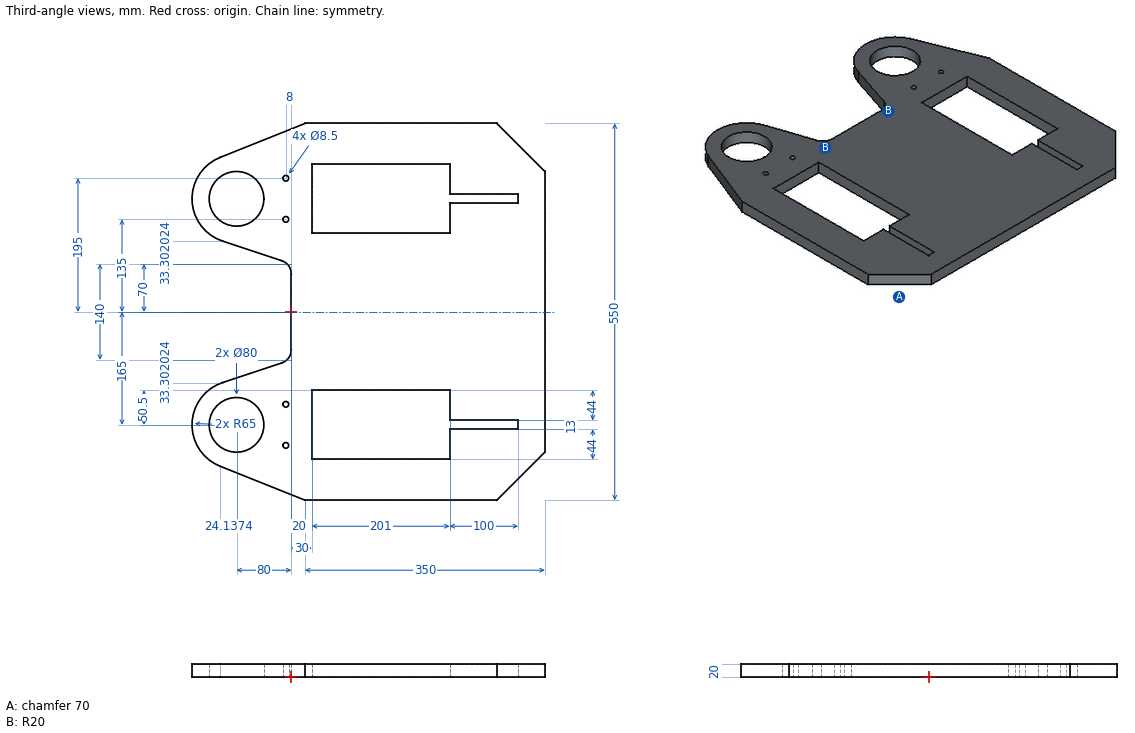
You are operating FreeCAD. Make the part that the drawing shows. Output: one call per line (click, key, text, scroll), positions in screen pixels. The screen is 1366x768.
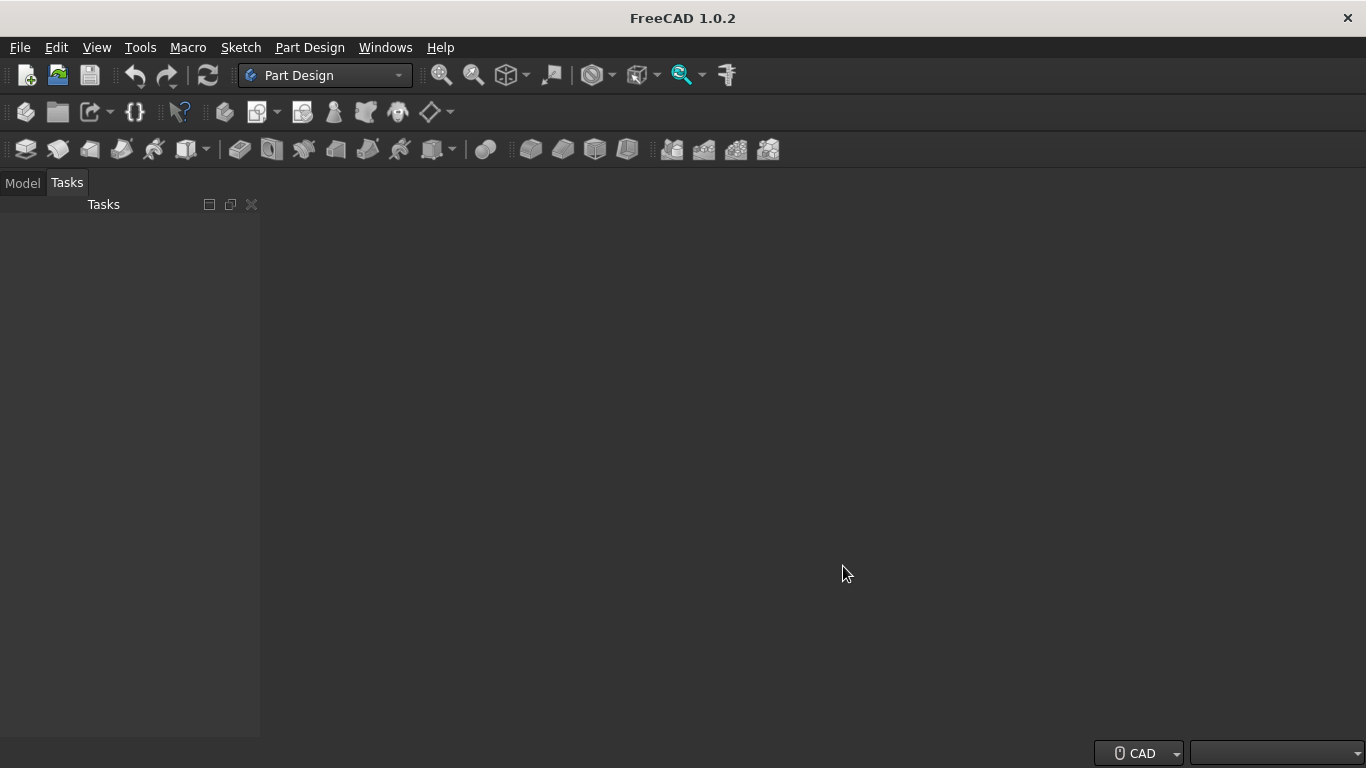
click(26, 76)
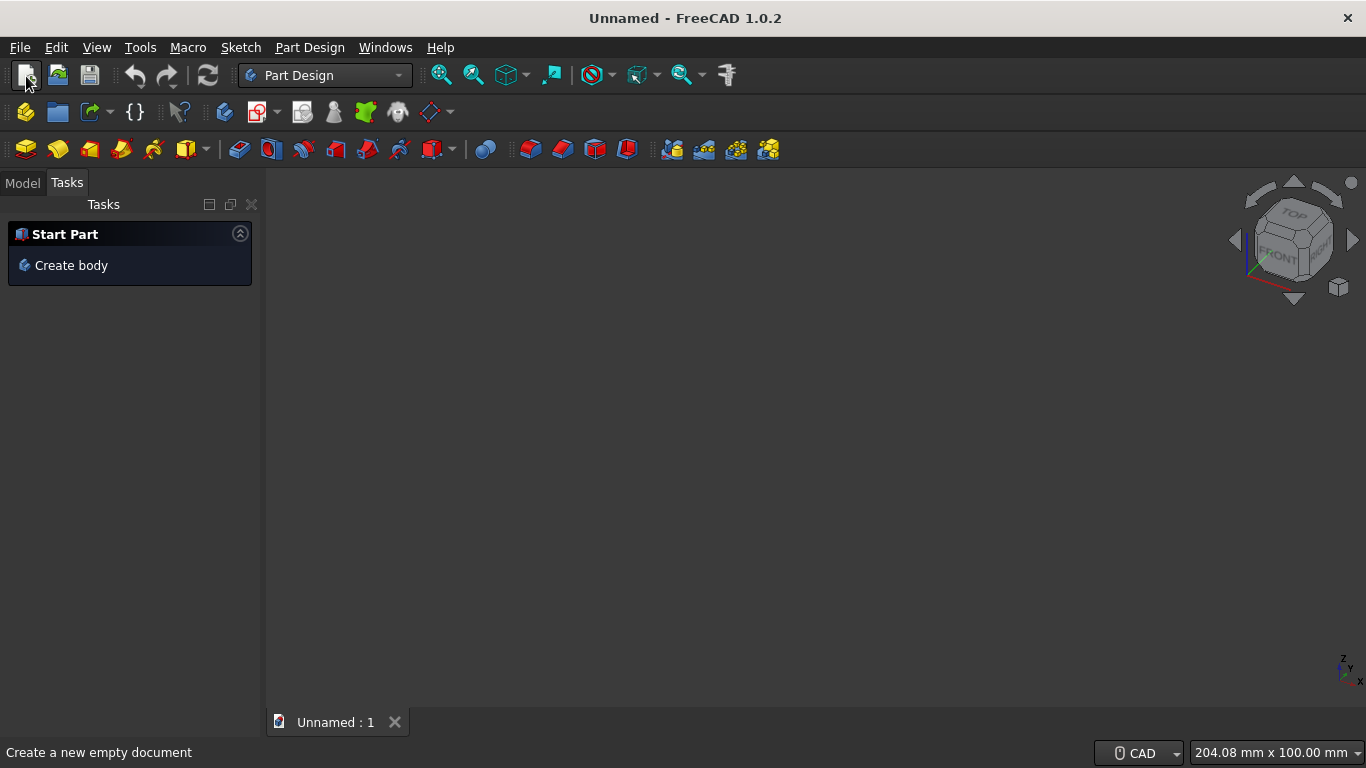
click(258, 112)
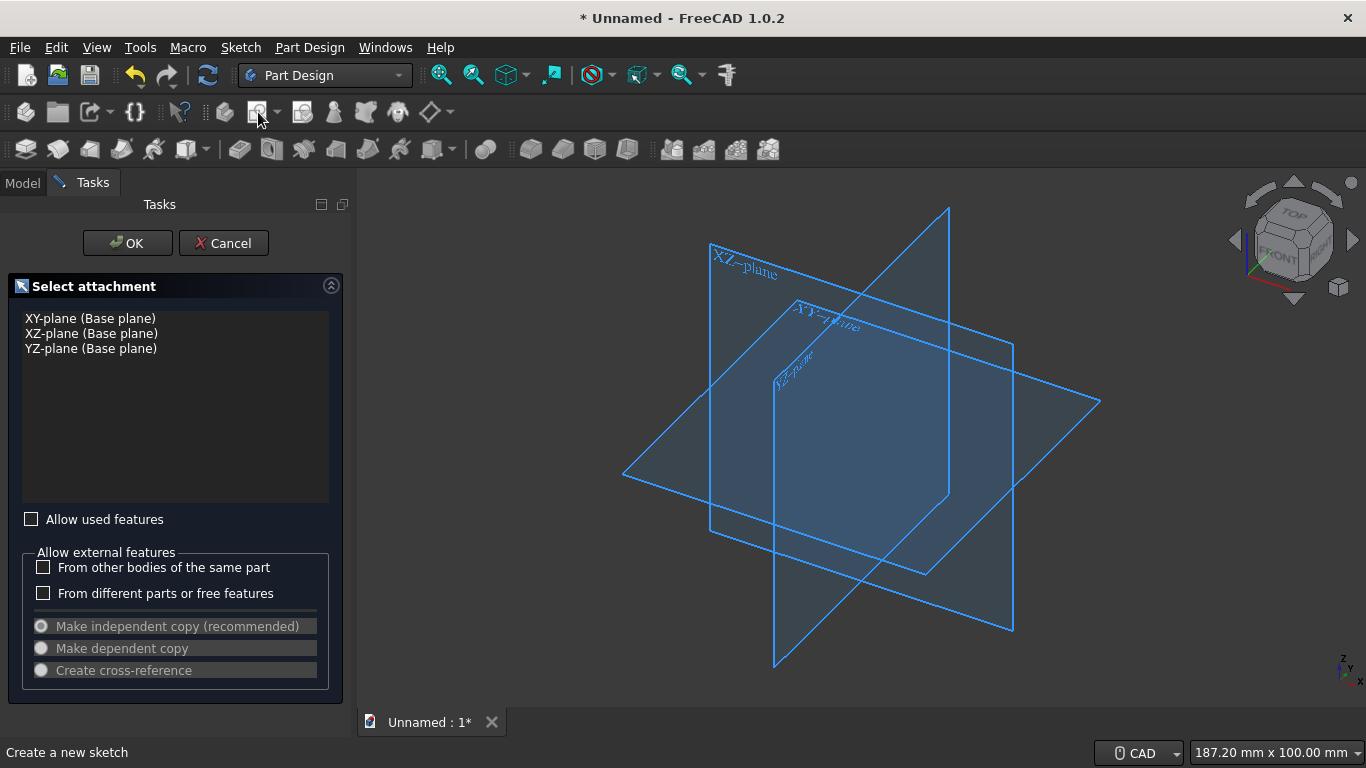
click(82, 318)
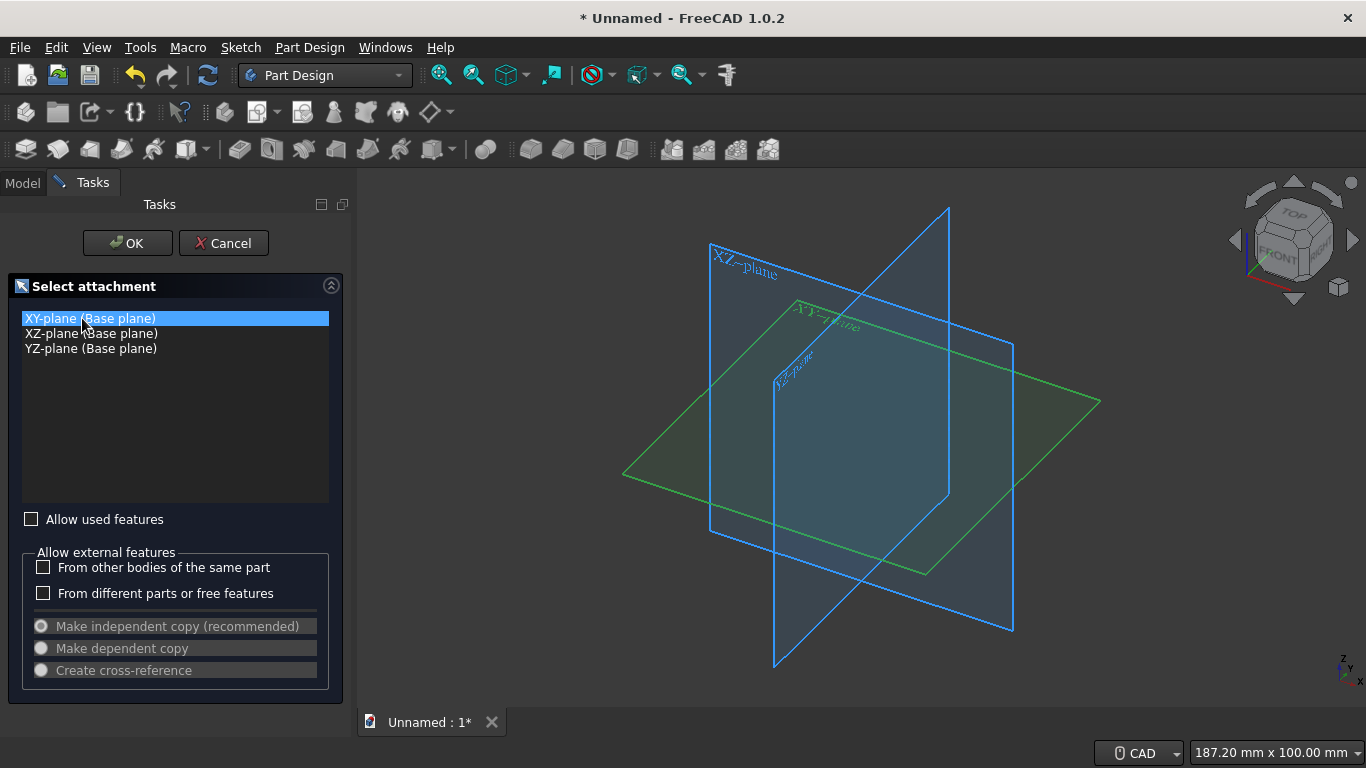
click(128, 243)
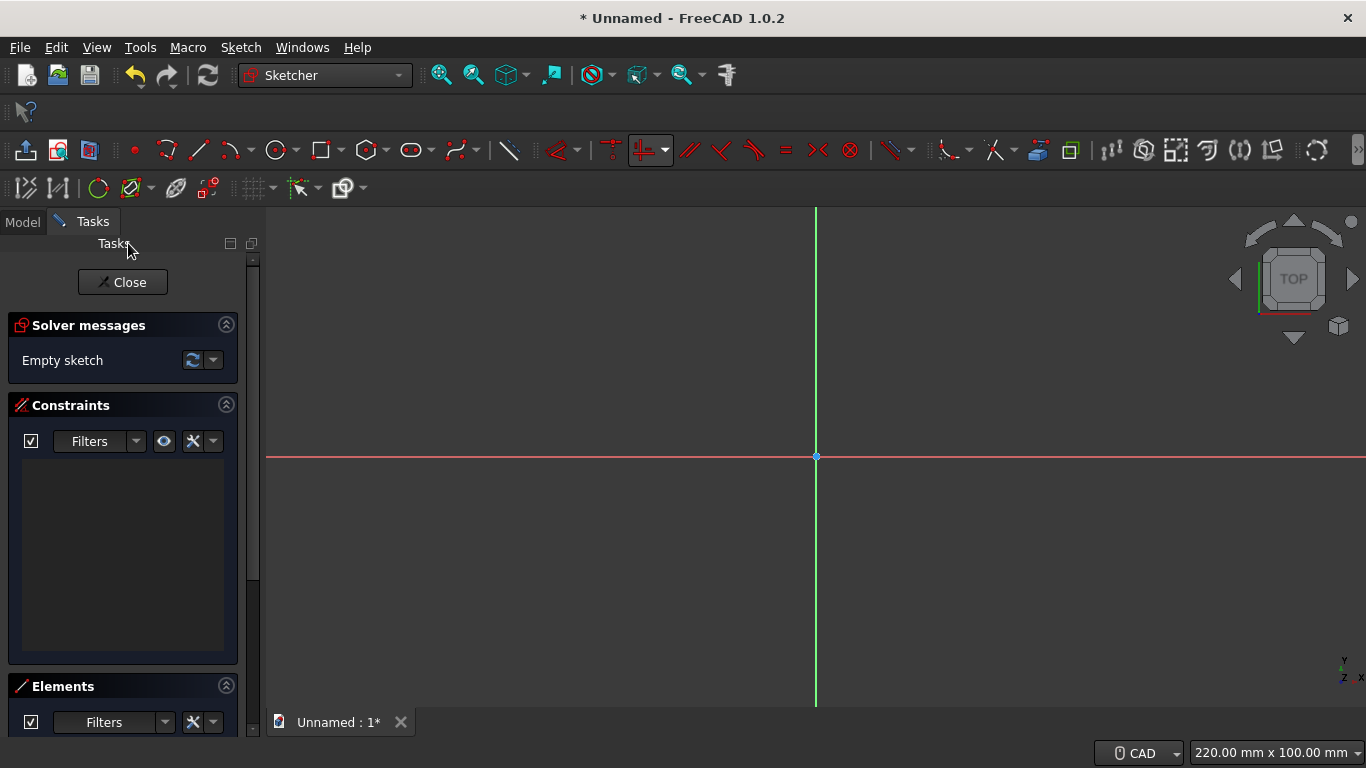
scroll(669, 457, down, 11)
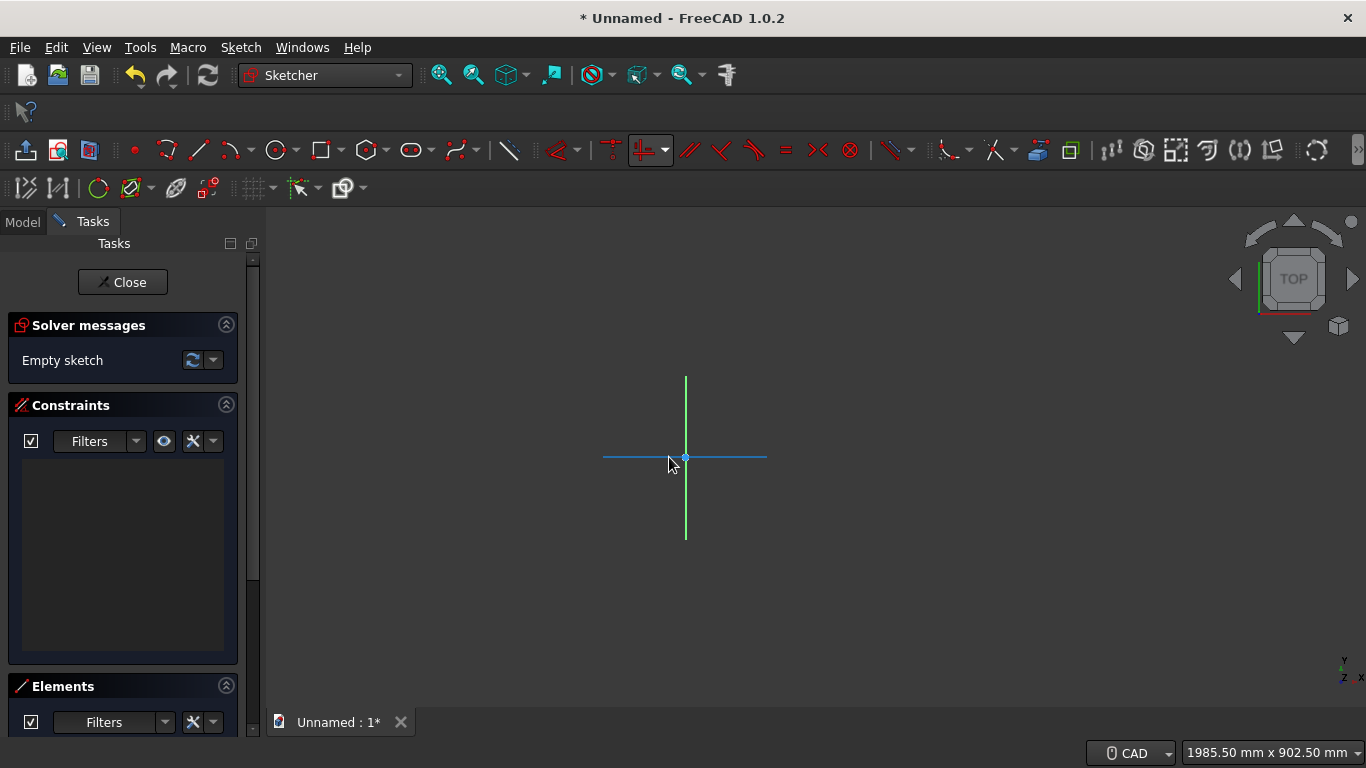
key(g)
key(m)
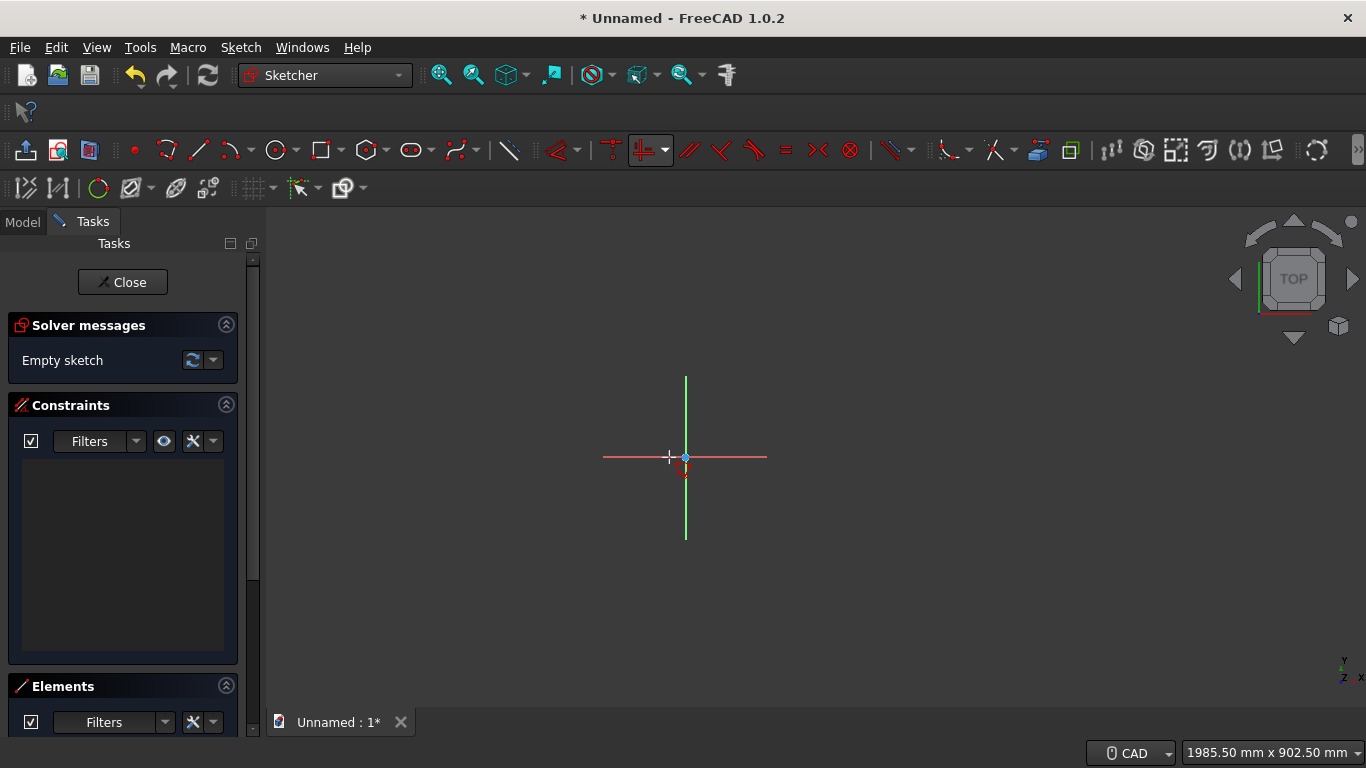
click(628, 582)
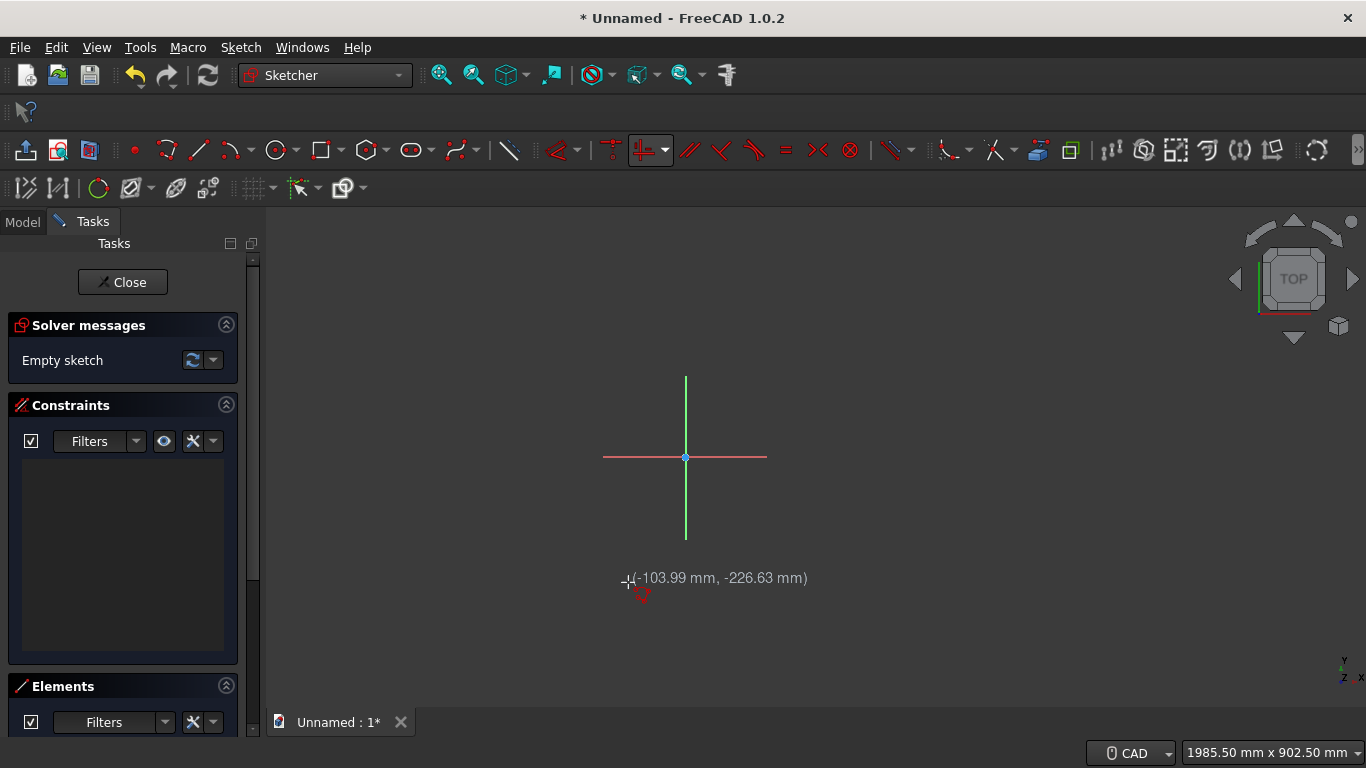
scroll(697, 610, up, 2)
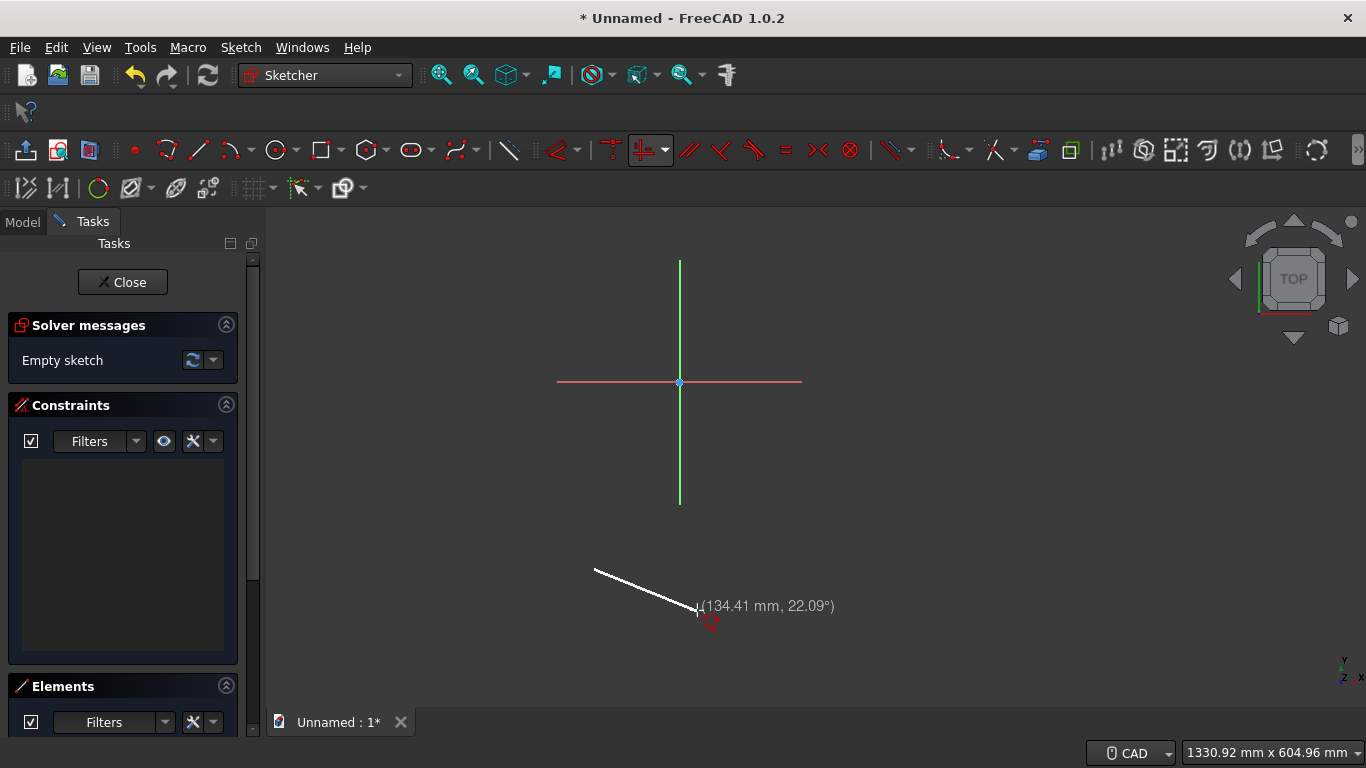
click(696, 609)
click(986, 609)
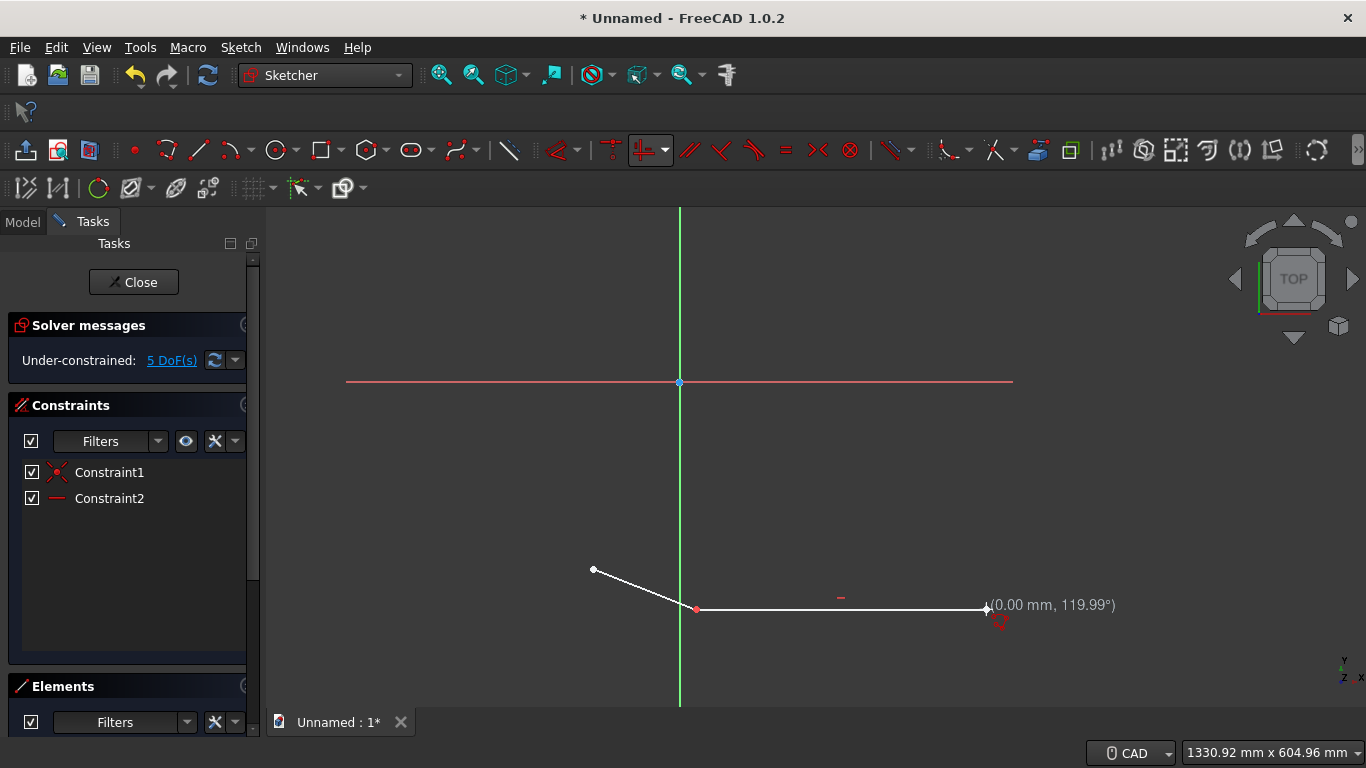
scroll(696, 609, down, 2)